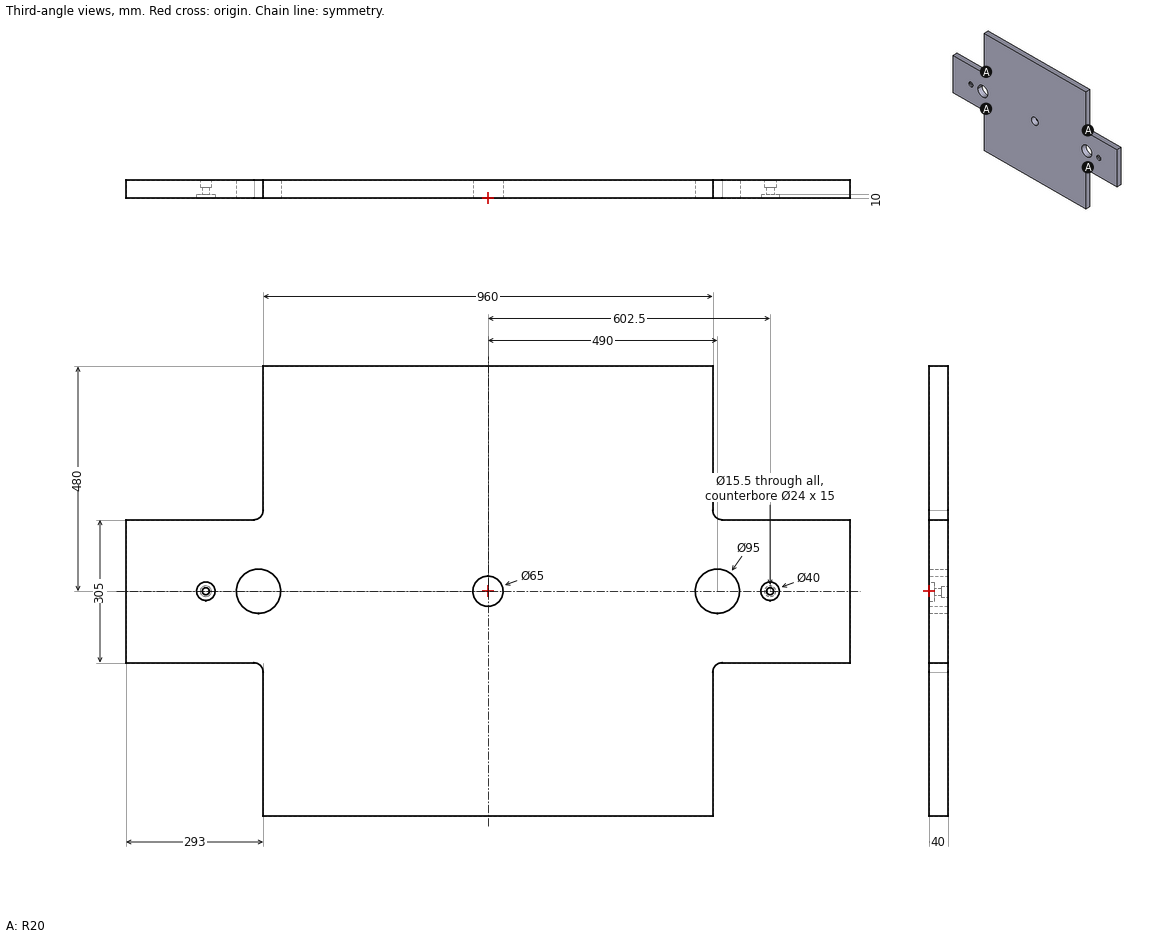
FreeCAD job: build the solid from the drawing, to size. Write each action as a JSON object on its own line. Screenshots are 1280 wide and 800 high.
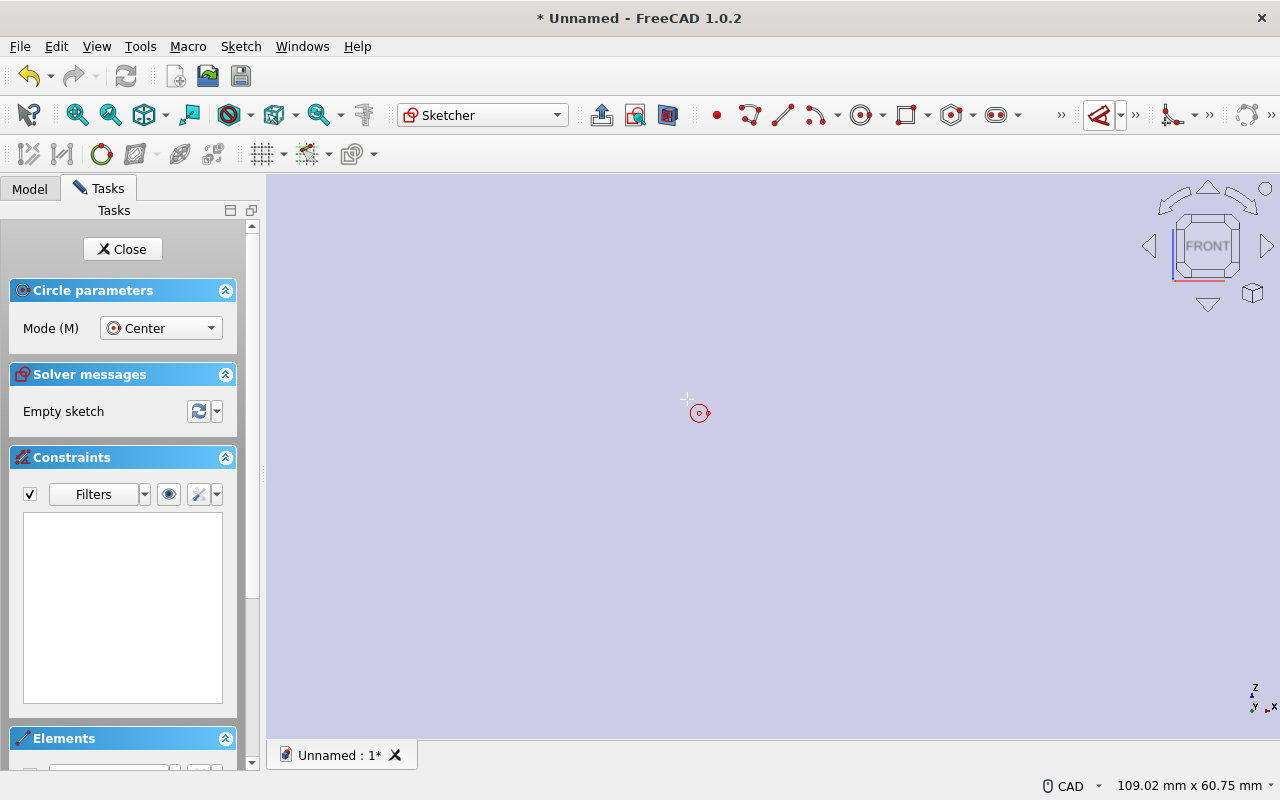
{"action": "left_click", "coordinate": [704, 456]}
{"action": "mouse_move", "coordinate": [836, 325]}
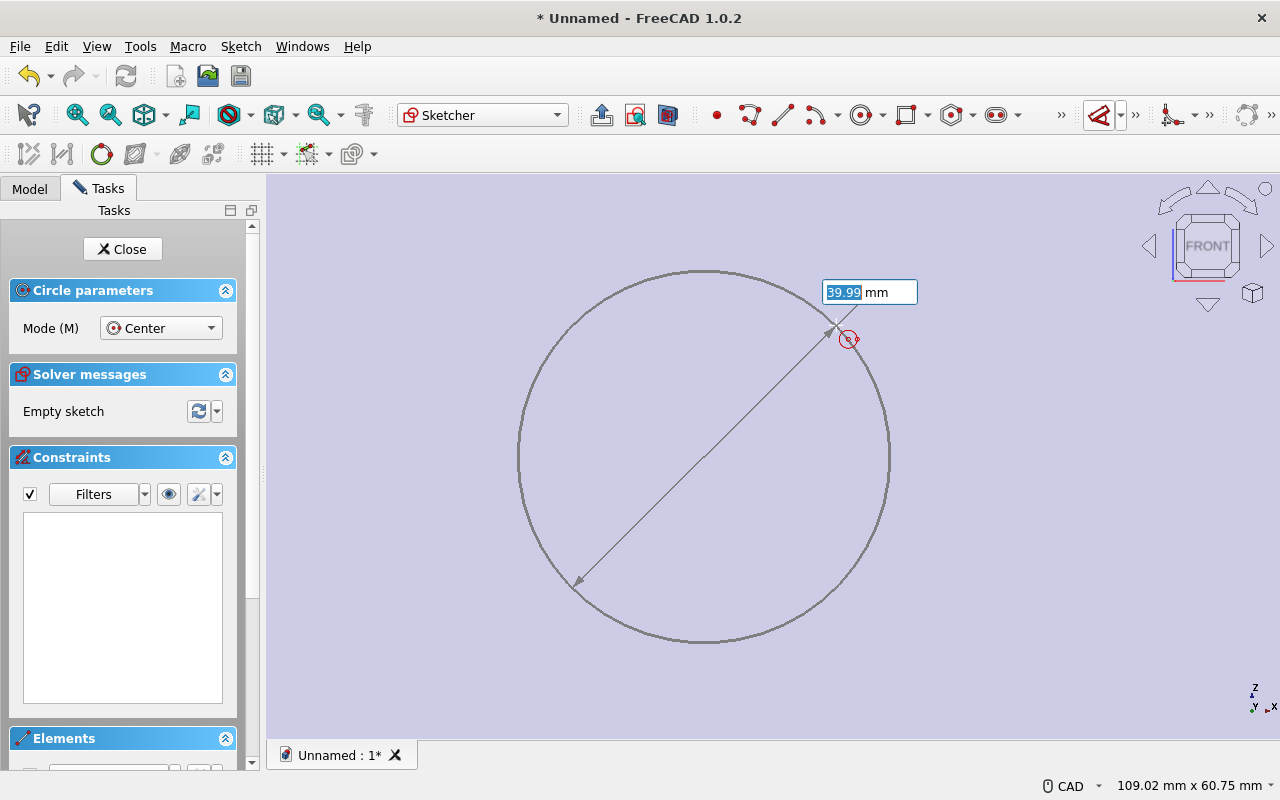
{"action": "type", "text": "40"}
{"action": "key", "text": "Return"}
{"action": "key", "text": "Escape"}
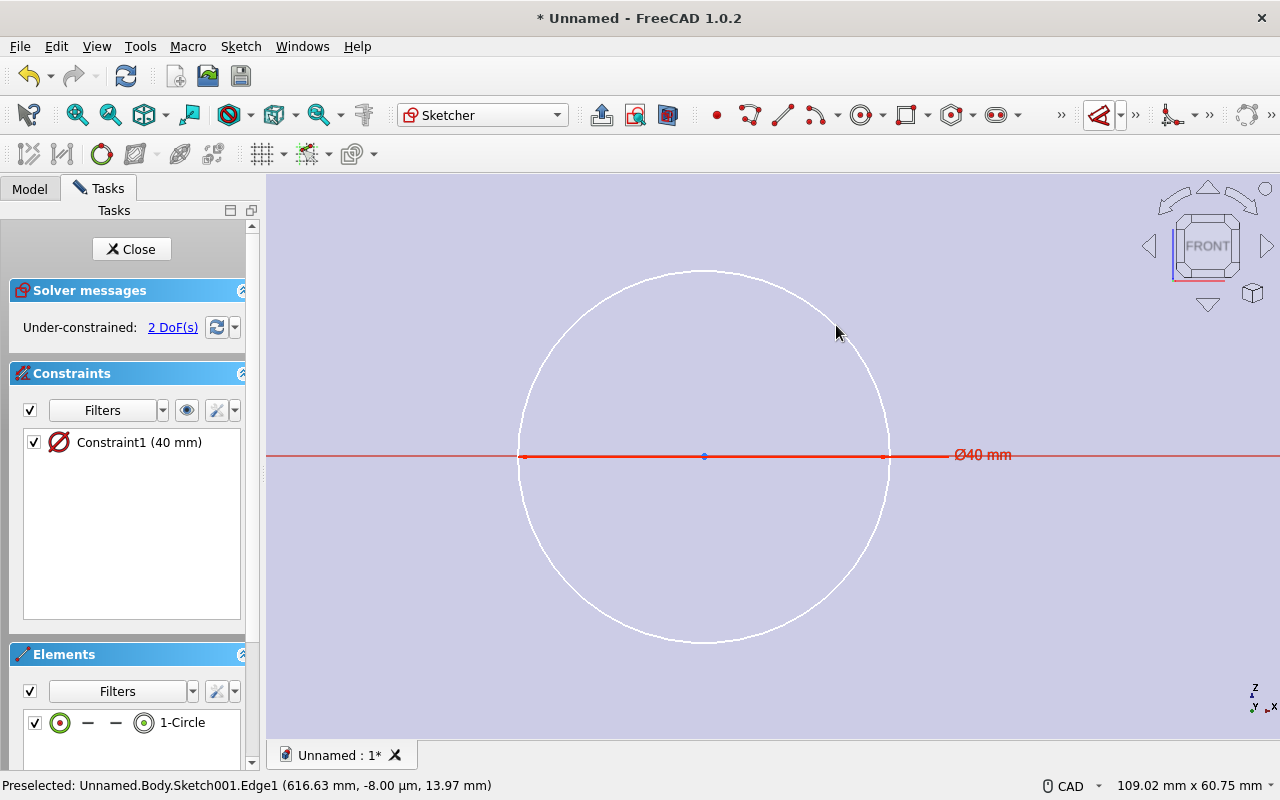
{"action": "left_click", "coordinate": [704, 457]}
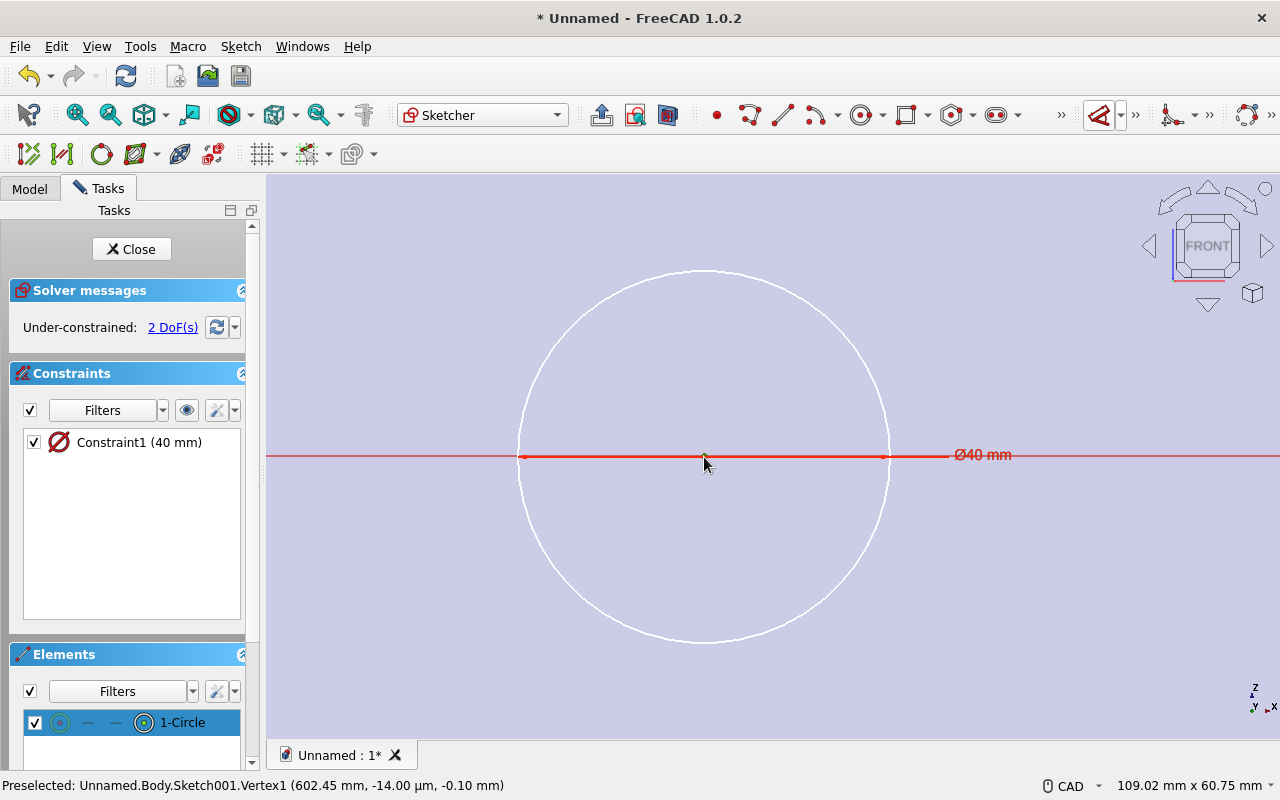
{"action": "left_click", "coordinate": [353, 456]}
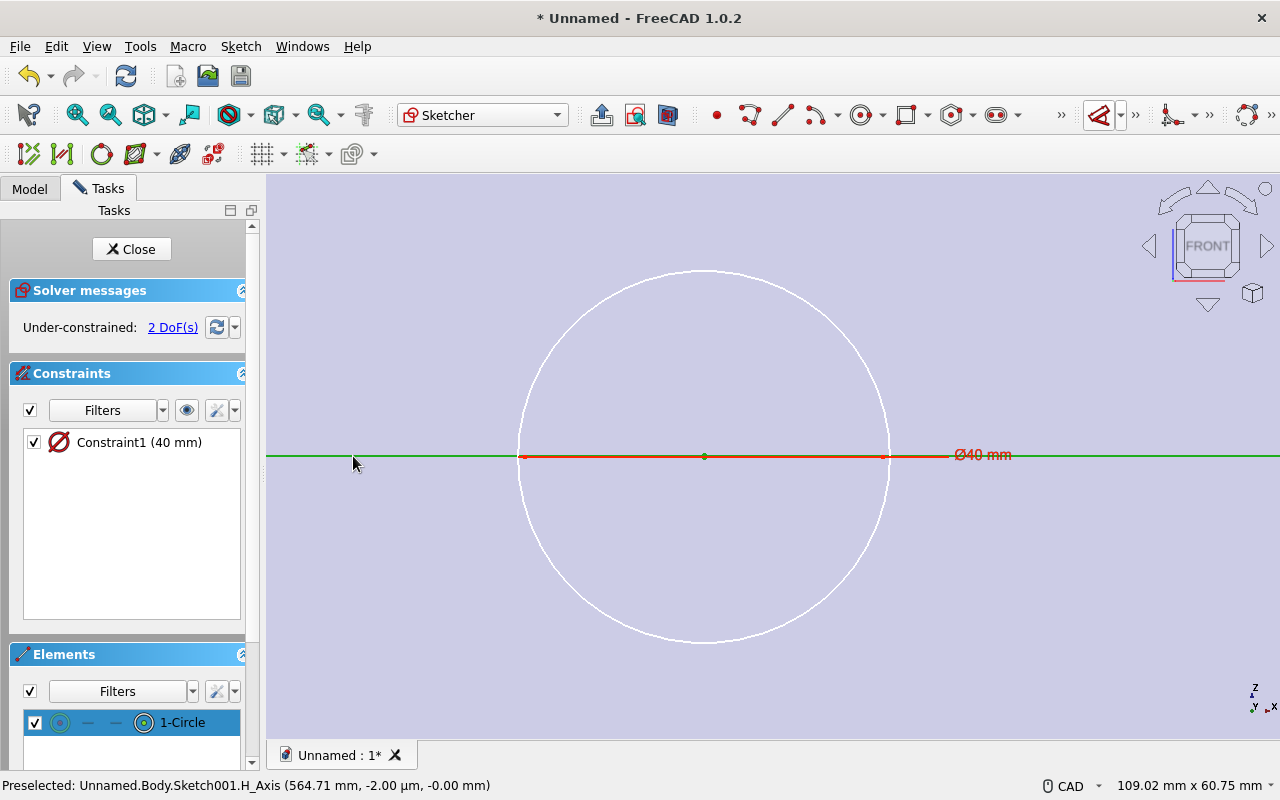
{"action": "key", "text": "c"}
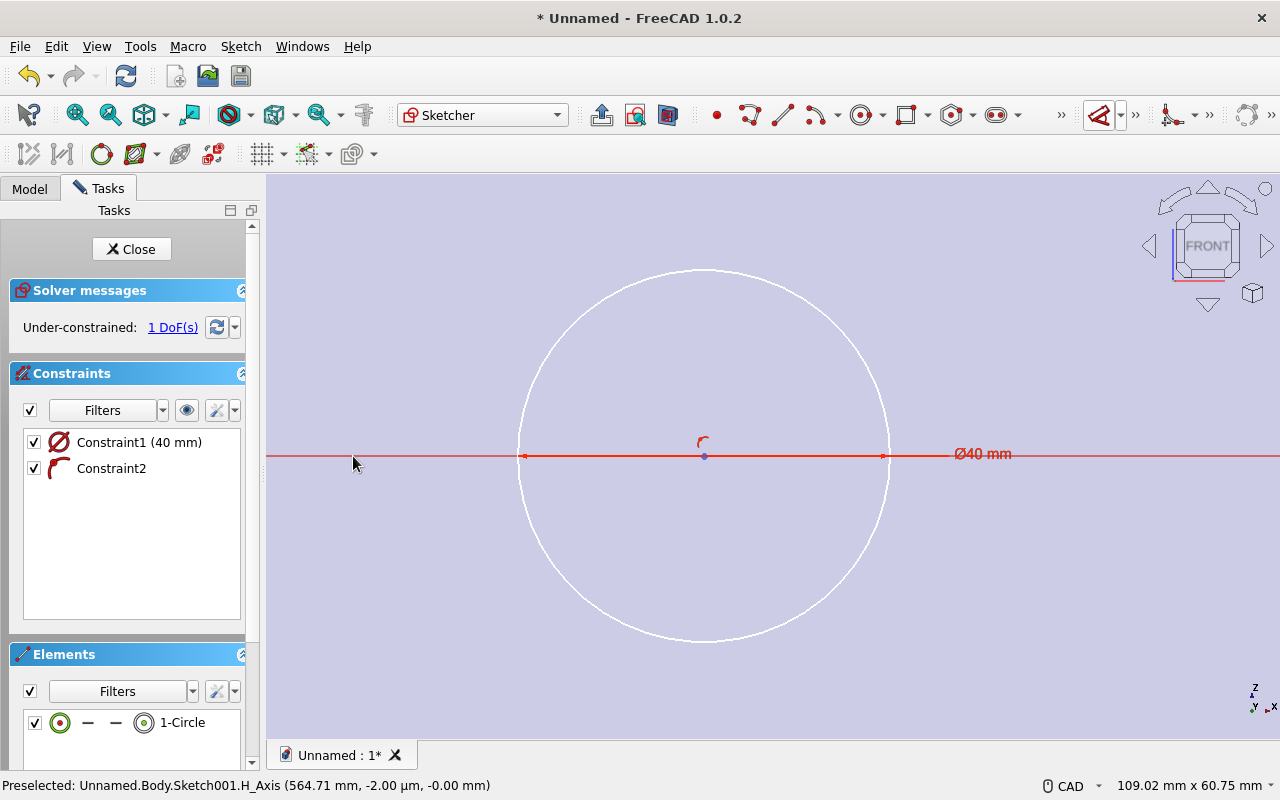
{"action": "left_click", "coordinate": [704, 456]}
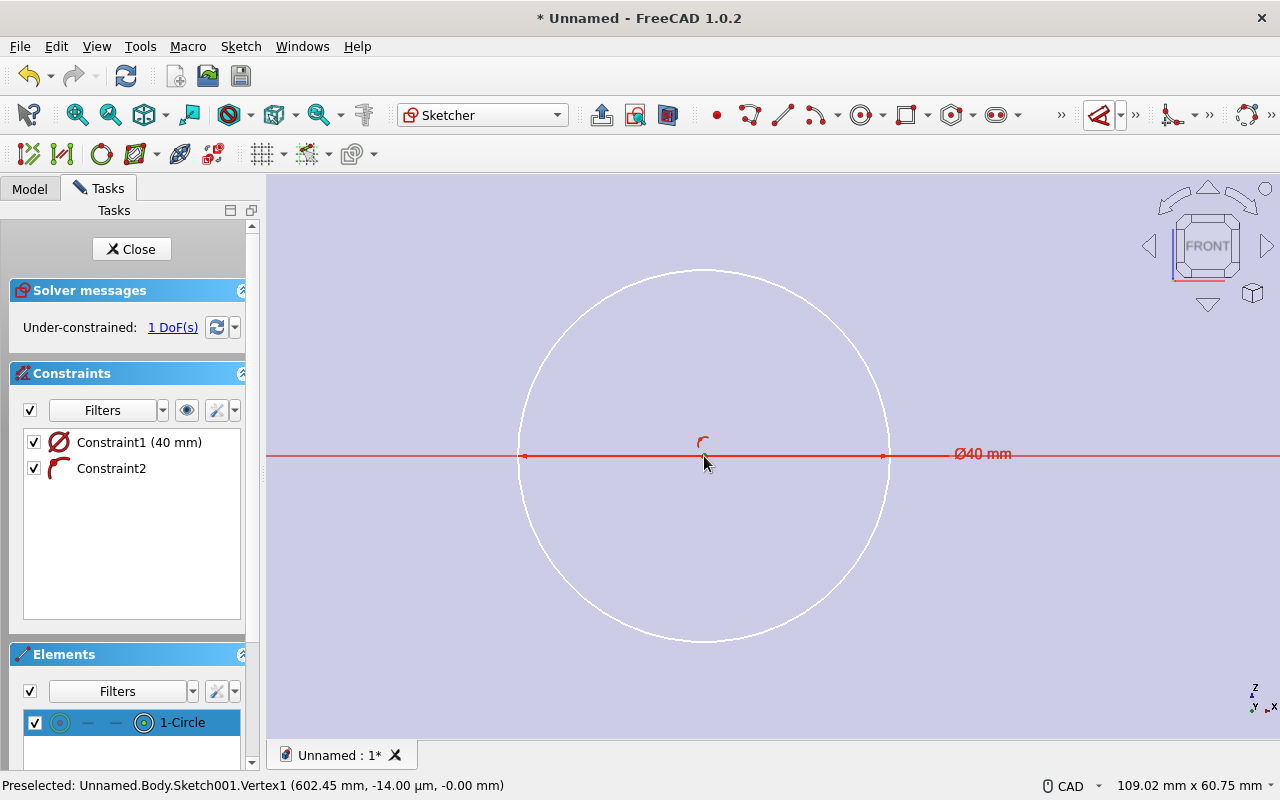
{"action": "key", "text": "l"}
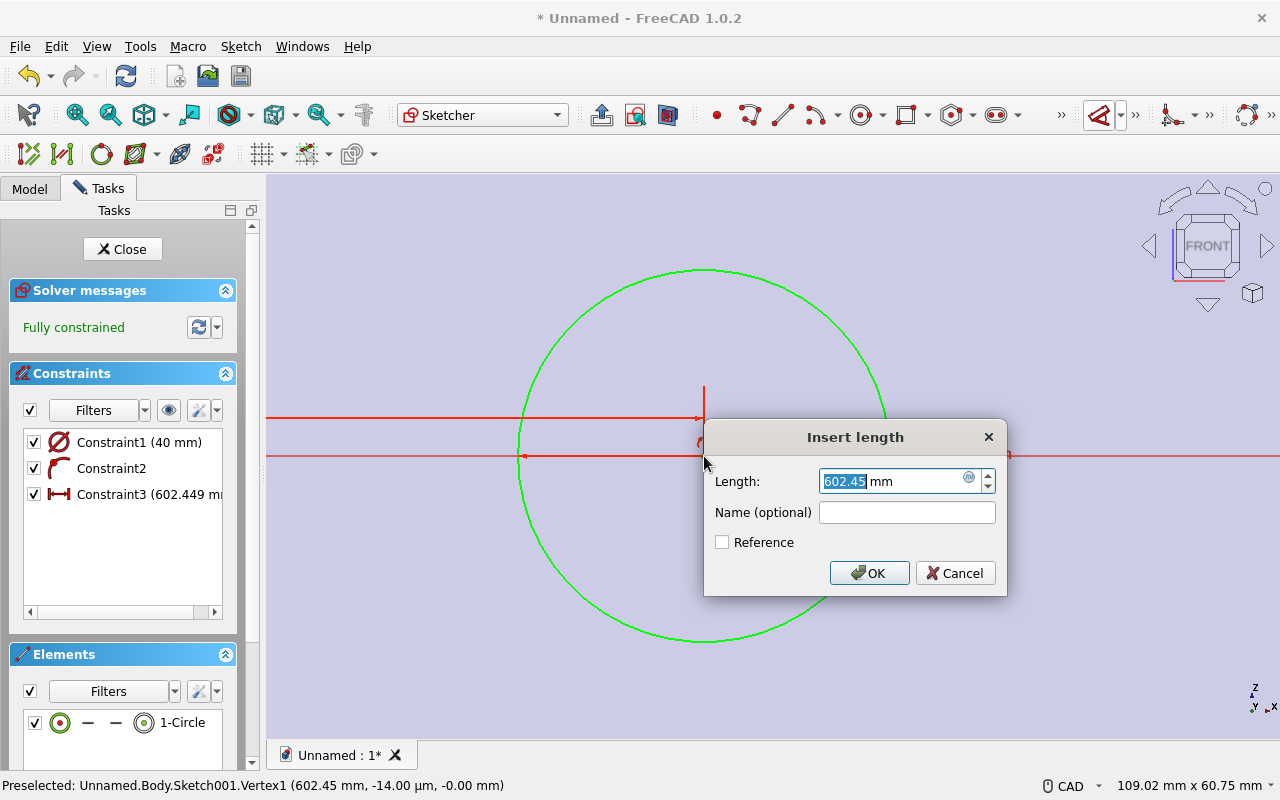
{"action": "type", "text": "602.5"}
{"action": "key", "text": "Return"}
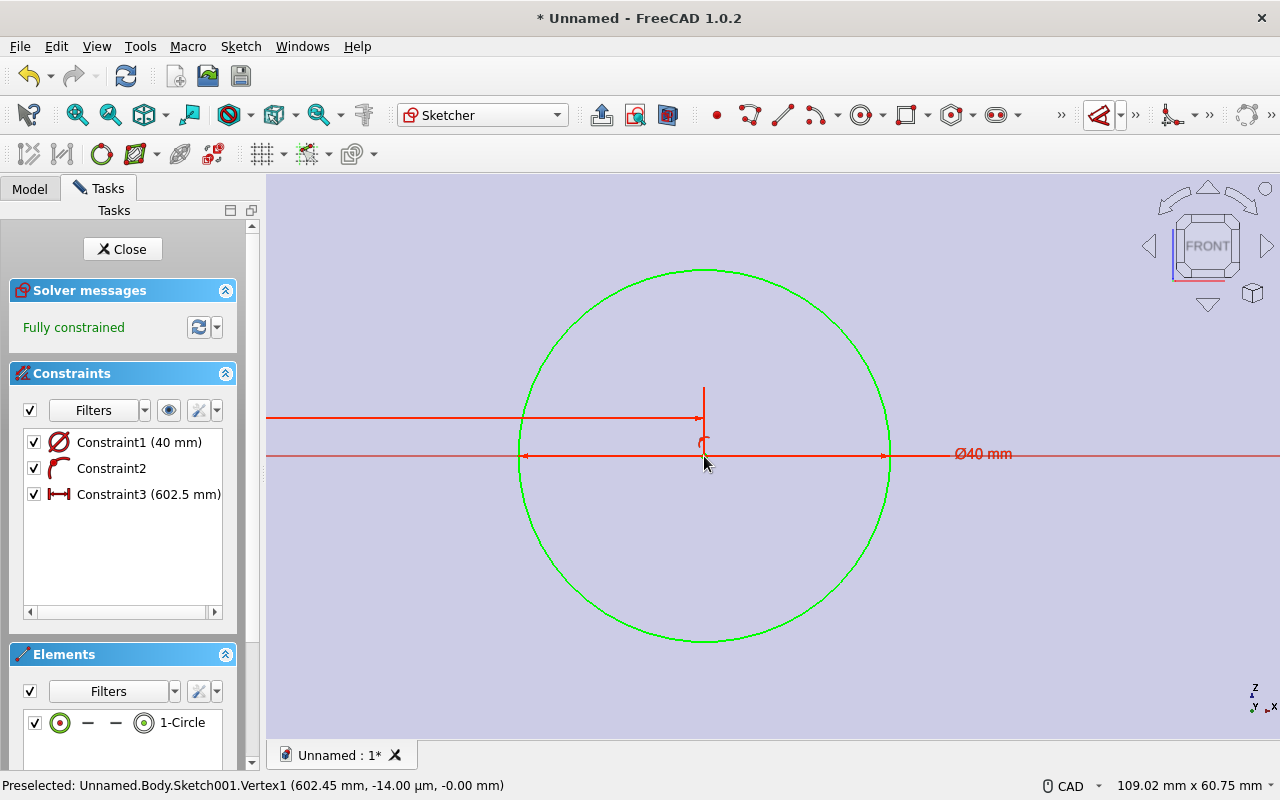
{"action": "left_click", "coordinate": [123, 249]}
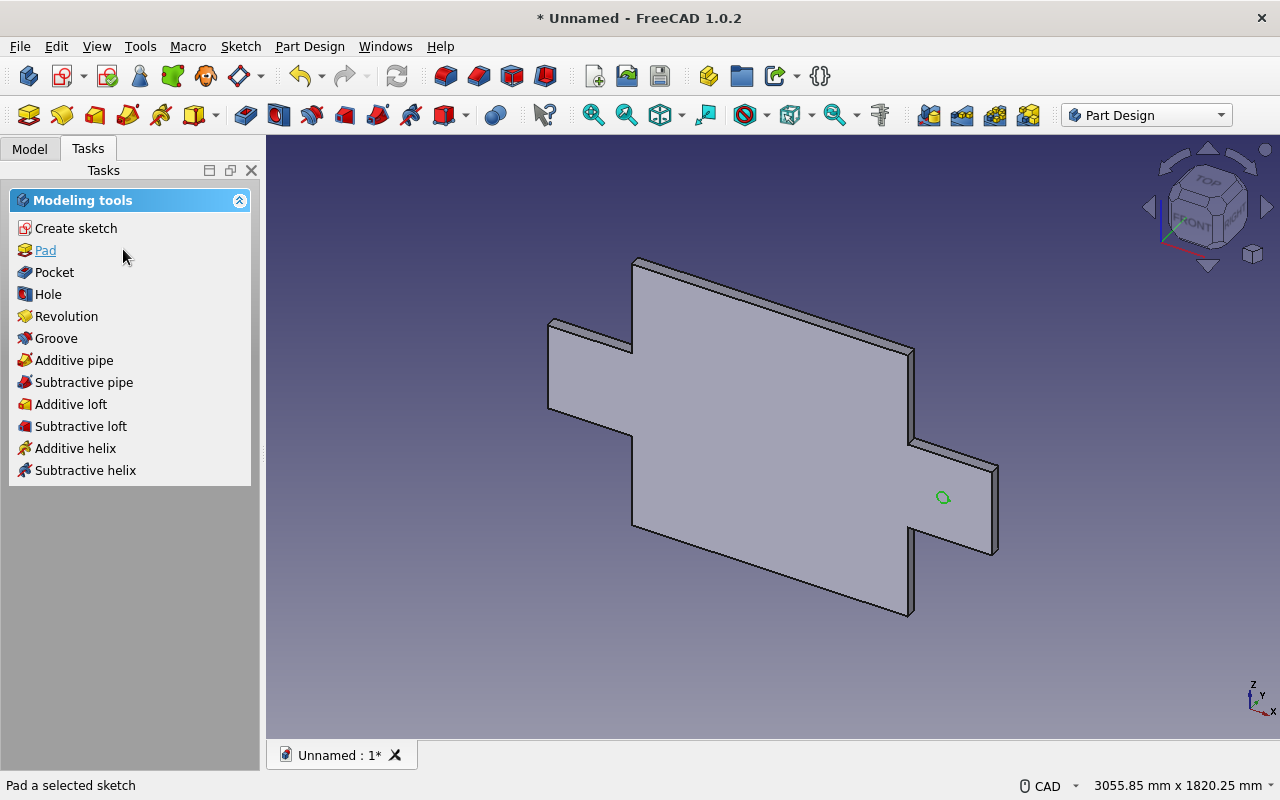
{"action": "left_click", "coordinate": [246, 116]}